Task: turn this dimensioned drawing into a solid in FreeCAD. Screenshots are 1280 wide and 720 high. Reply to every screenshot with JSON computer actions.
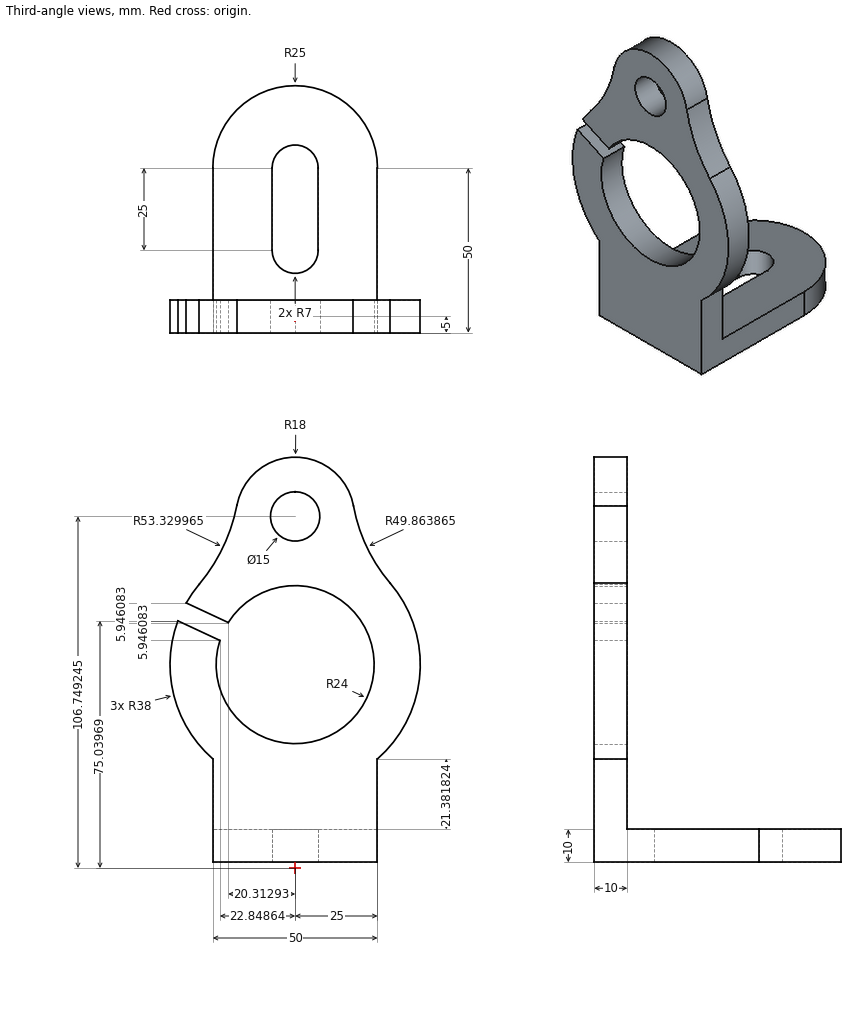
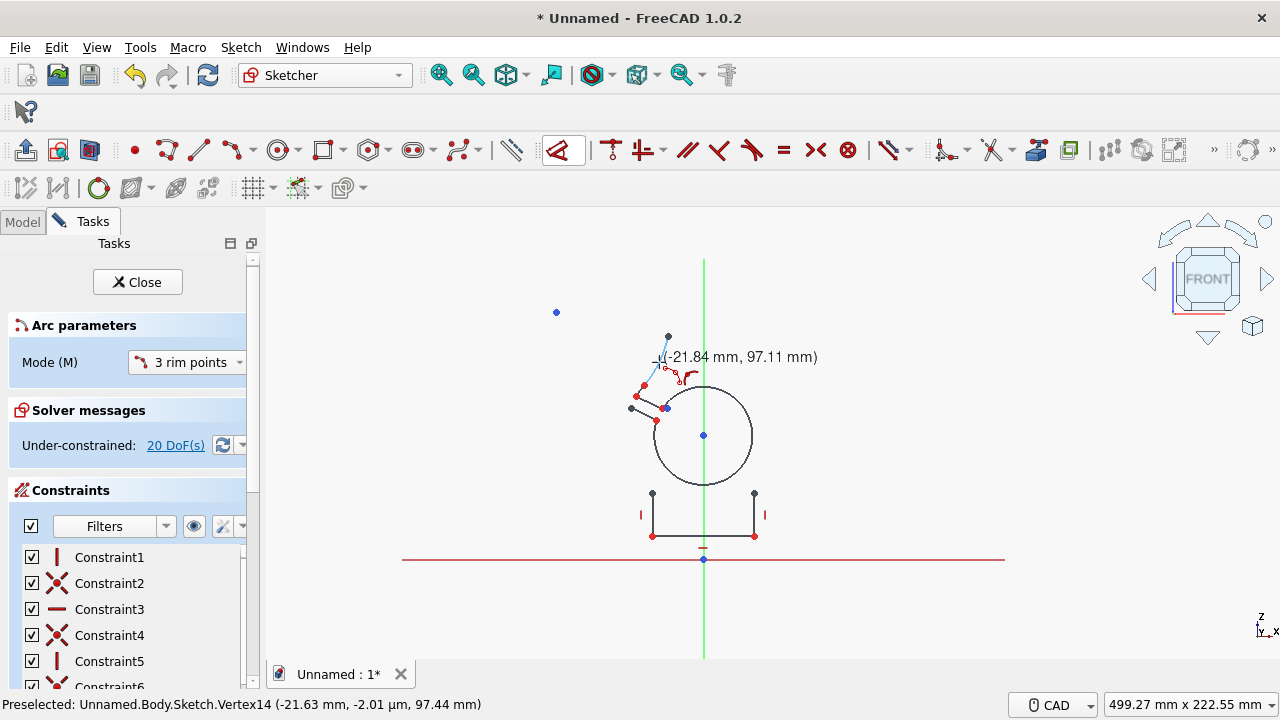
{"action": "left_click", "coordinate": [668, 337]}
{"action": "left_click", "coordinate": [740, 336]}
{"action": "left_click", "coordinate": [723, 312]}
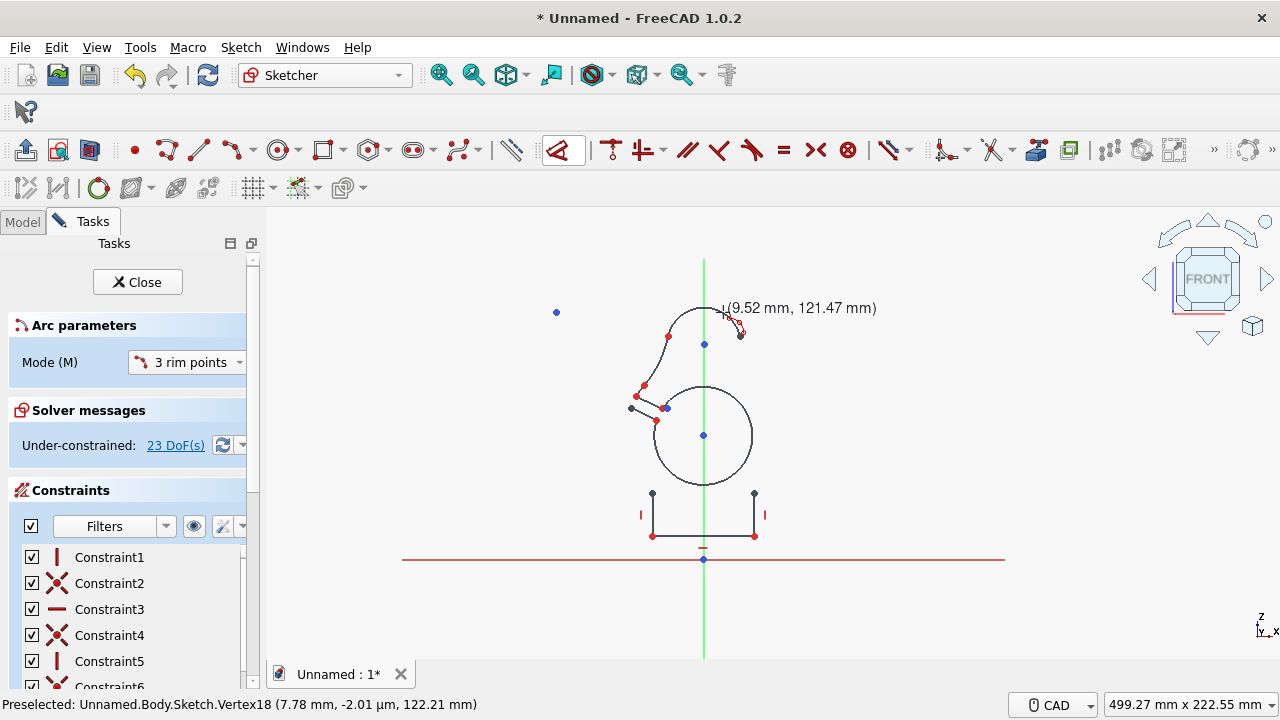
{"action": "left_click", "coordinate": [740, 337]}
{"action": "left_click", "coordinate": [762, 384]}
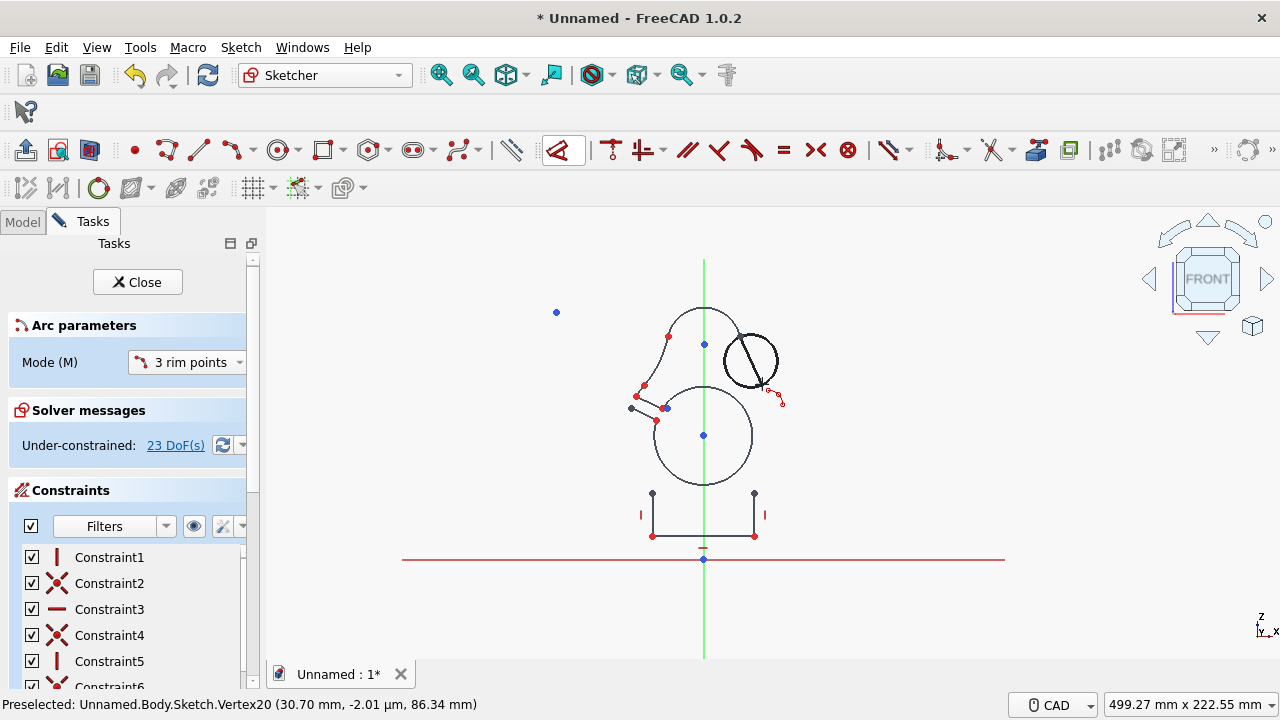
{"action": "scroll", "coordinate": [748, 362], "scroll_direction": "up", "scroll_amount": 8}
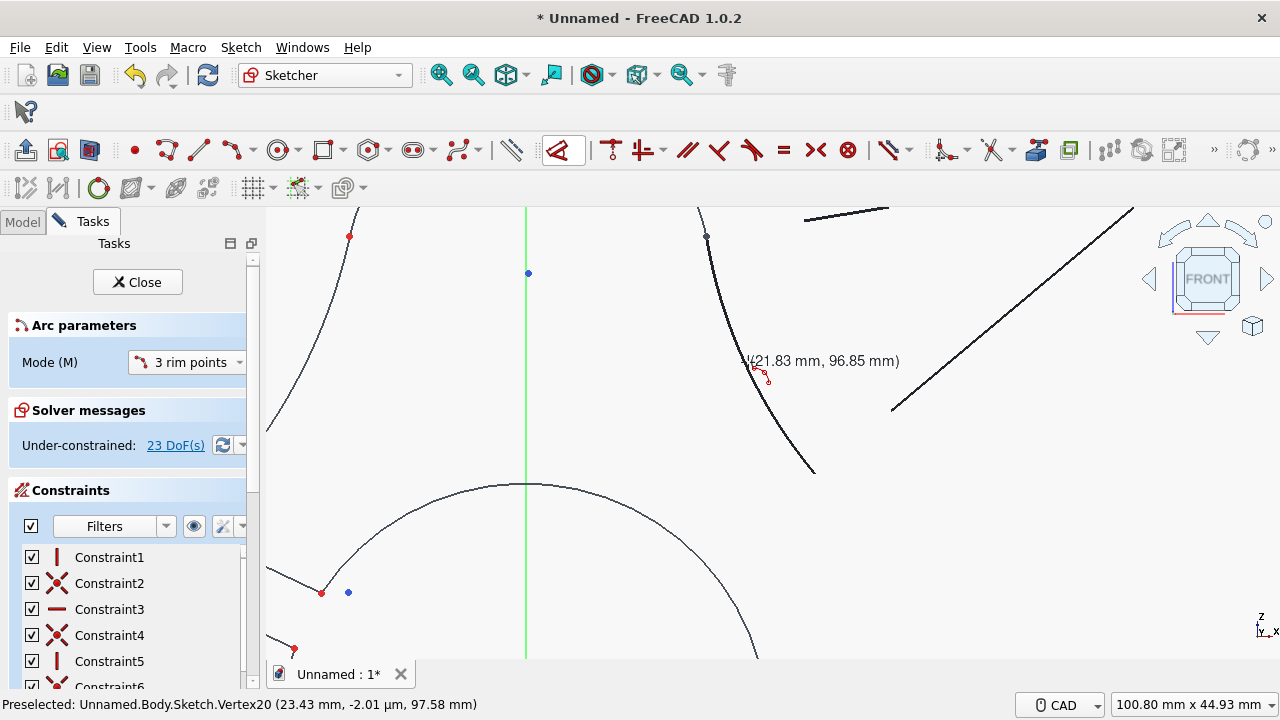
{"action": "left_click", "coordinate": [745, 359]}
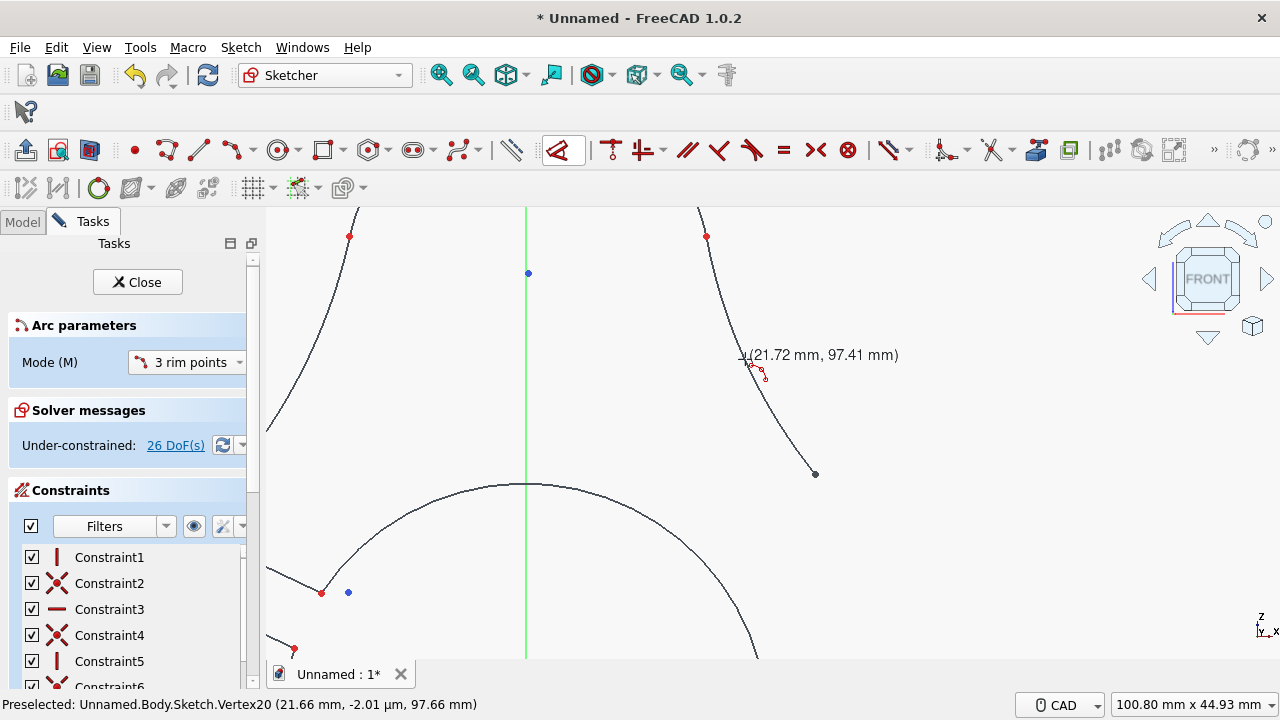
{"action": "scroll", "coordinate": [748, 362], "scroll_direction": "down", "scroll_amount": 8}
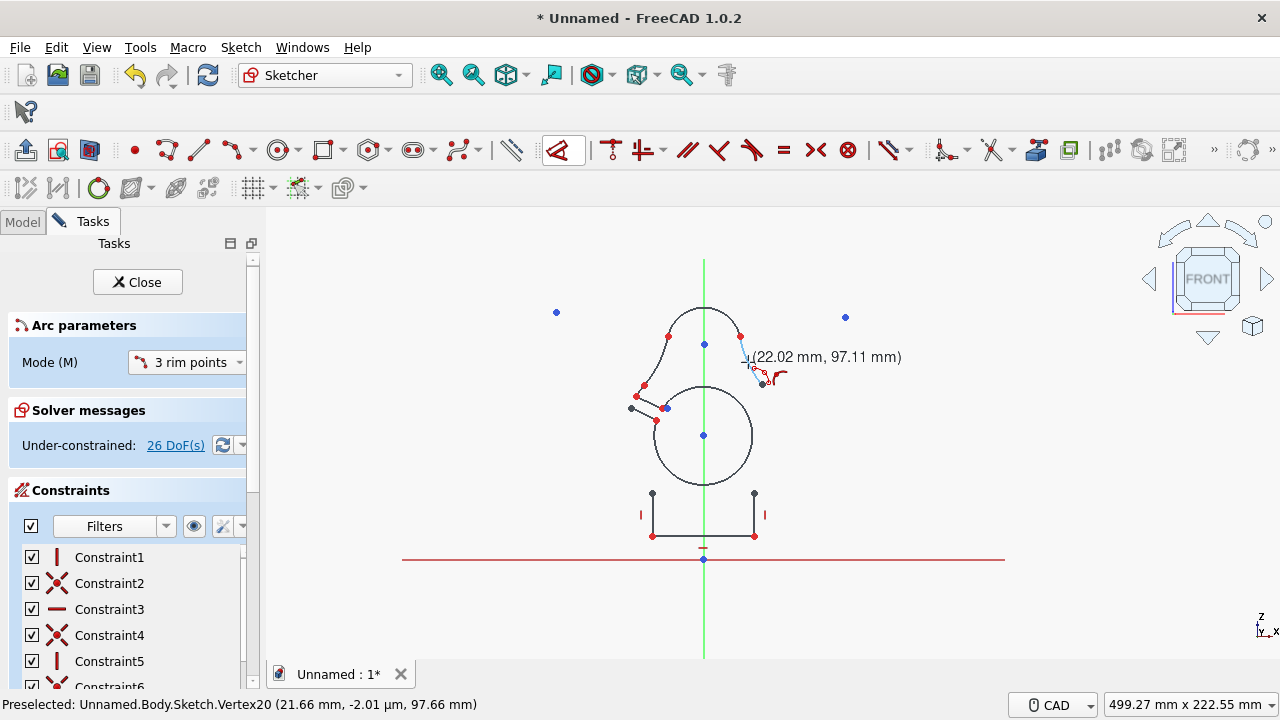
{"action": "left_click", "coordinate": [762, 385]}
{"action": "left_click", "coordinate": [754, 493]}
{"action": "left_click", "coordinate": [781, 440]}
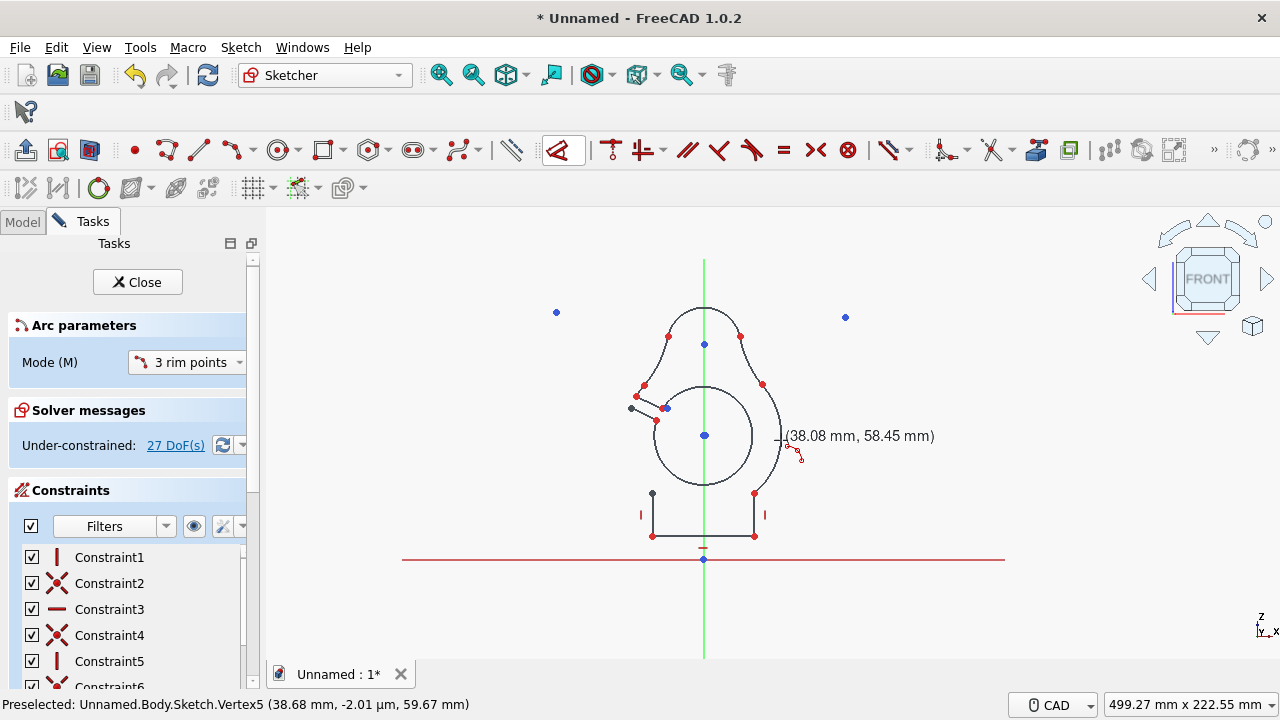
{"action": "left_click", "coordinate": [653, 493]}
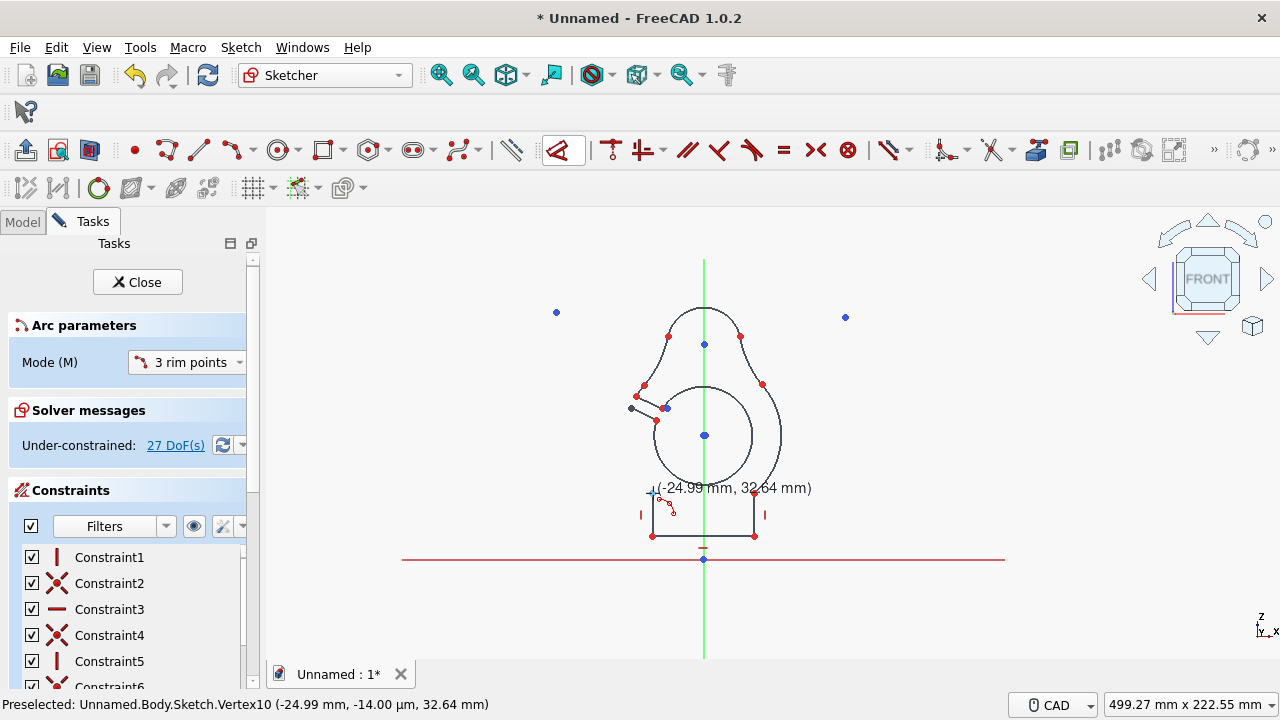
{"action": "scroll", "coordinate": [631, 407], "scroll_direction": "up", "scroll_amount": 2}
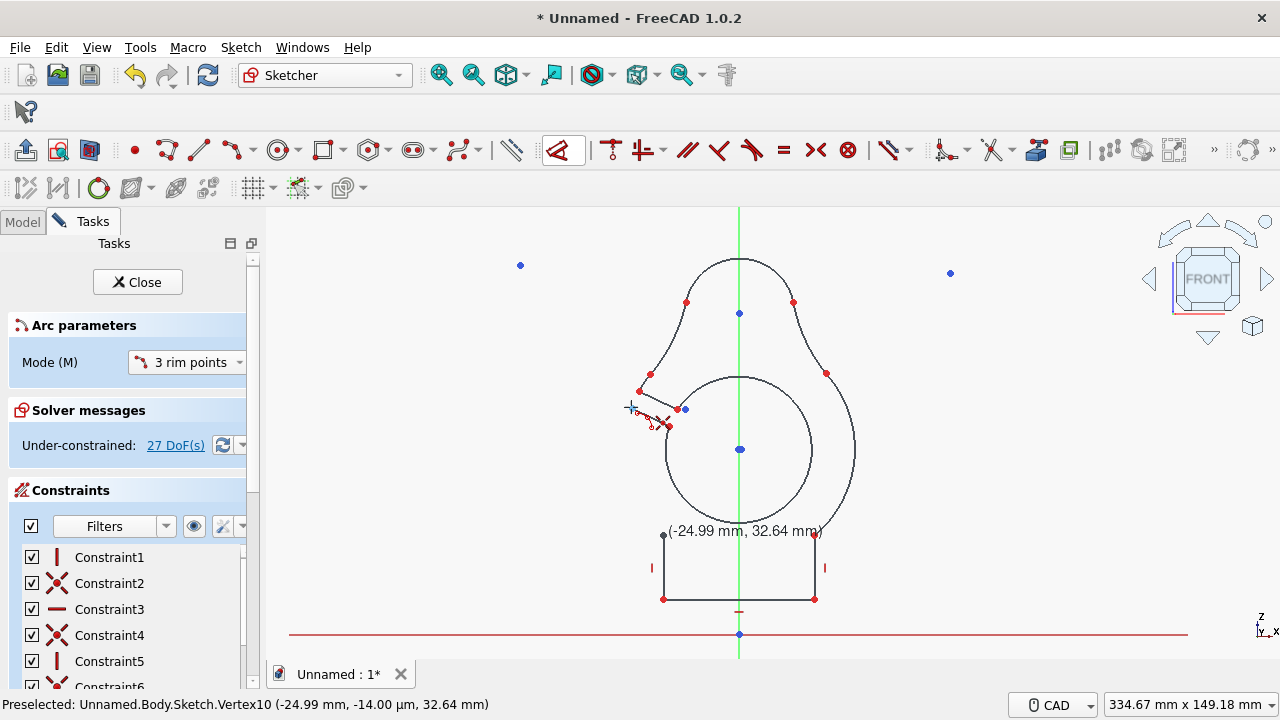
{"action": "left_click", "coordinate": [632, 409]}
{"action": "left_click", "coordinate": [628, 476]}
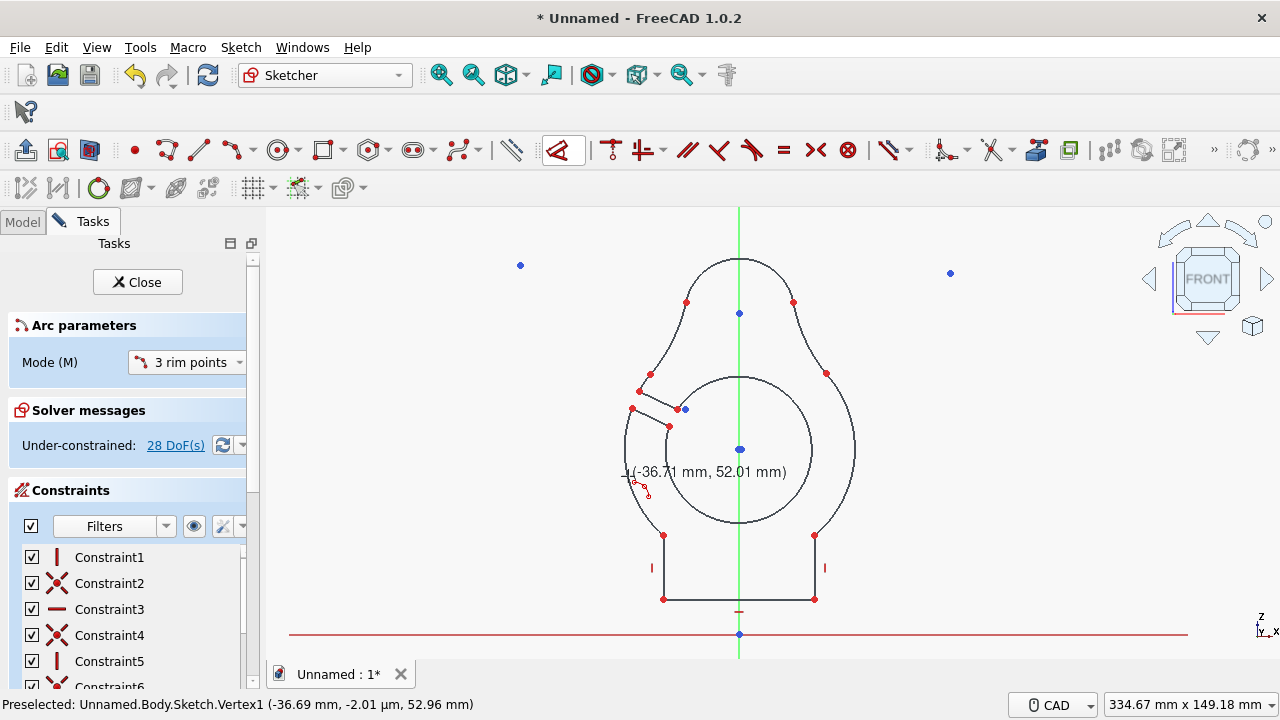
{"action": "left_click", "coordinate": [278, 150]}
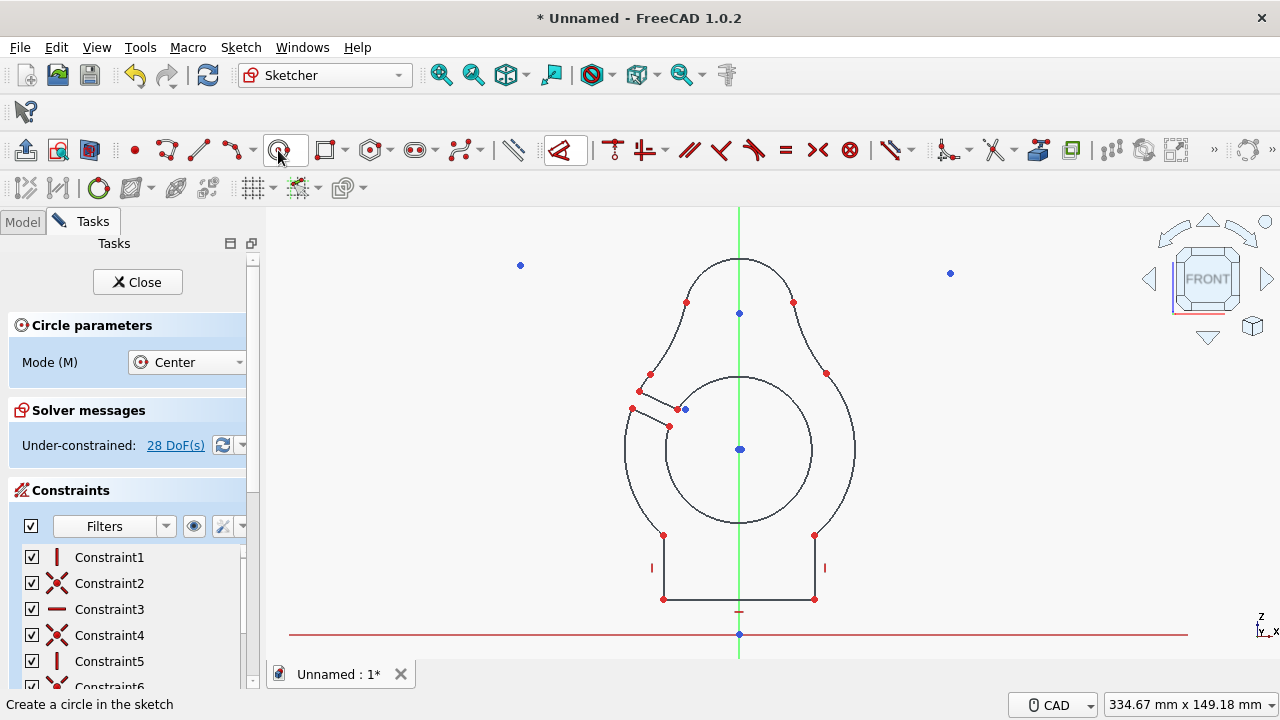
{"action": "left_click", "coordinate": [739, 311]}
{"action": "mouse_move", "coordinate": [755, 295]}